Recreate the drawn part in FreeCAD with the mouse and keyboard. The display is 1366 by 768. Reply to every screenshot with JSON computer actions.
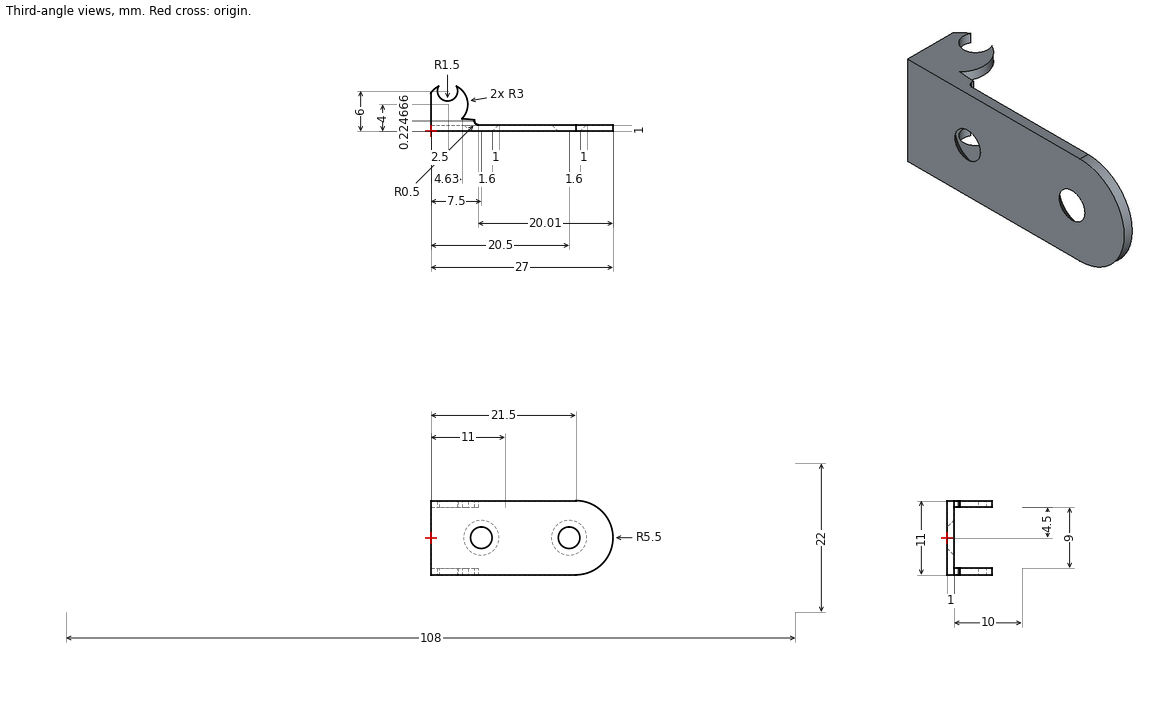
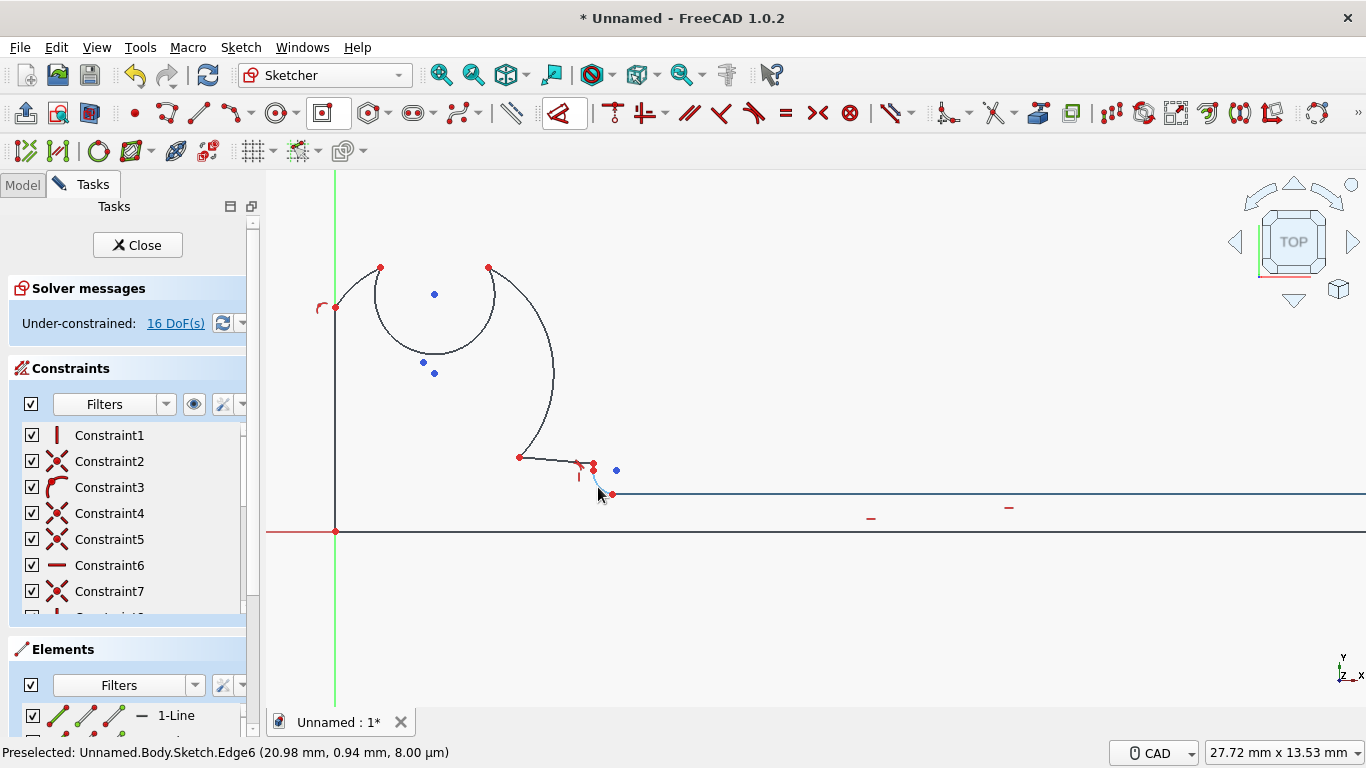
{"action": "left_click", "coordinate": [599, 486]}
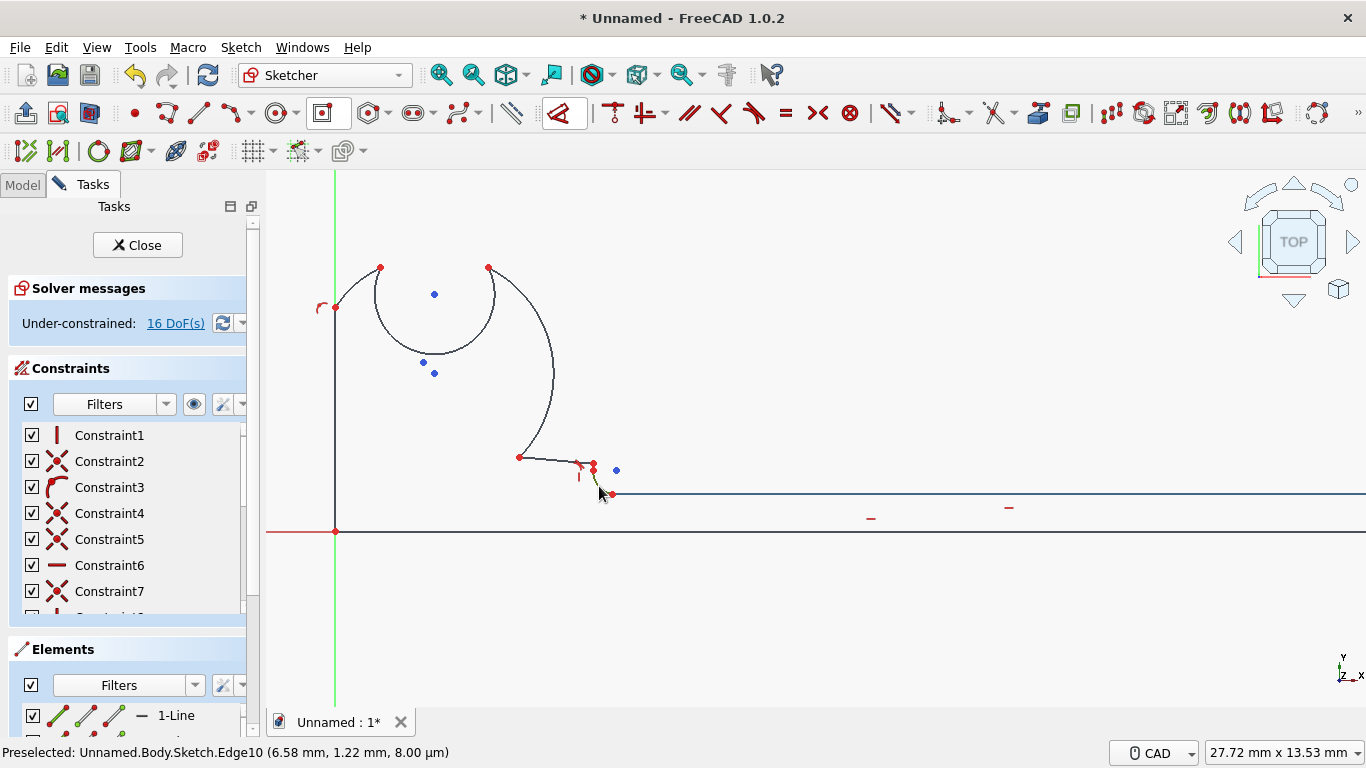
{"action": "key", "text": "t"}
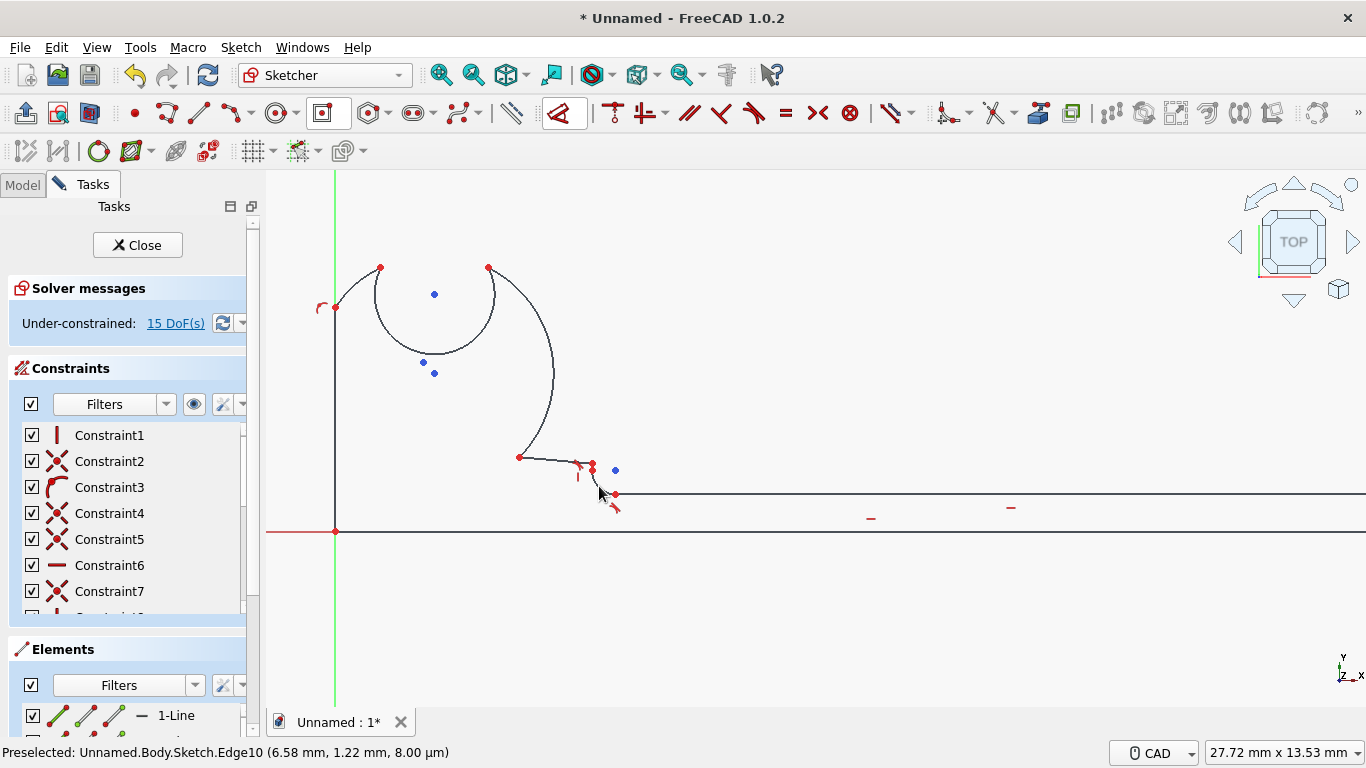
{"action": "left_click", "coordinate": [551, 399]}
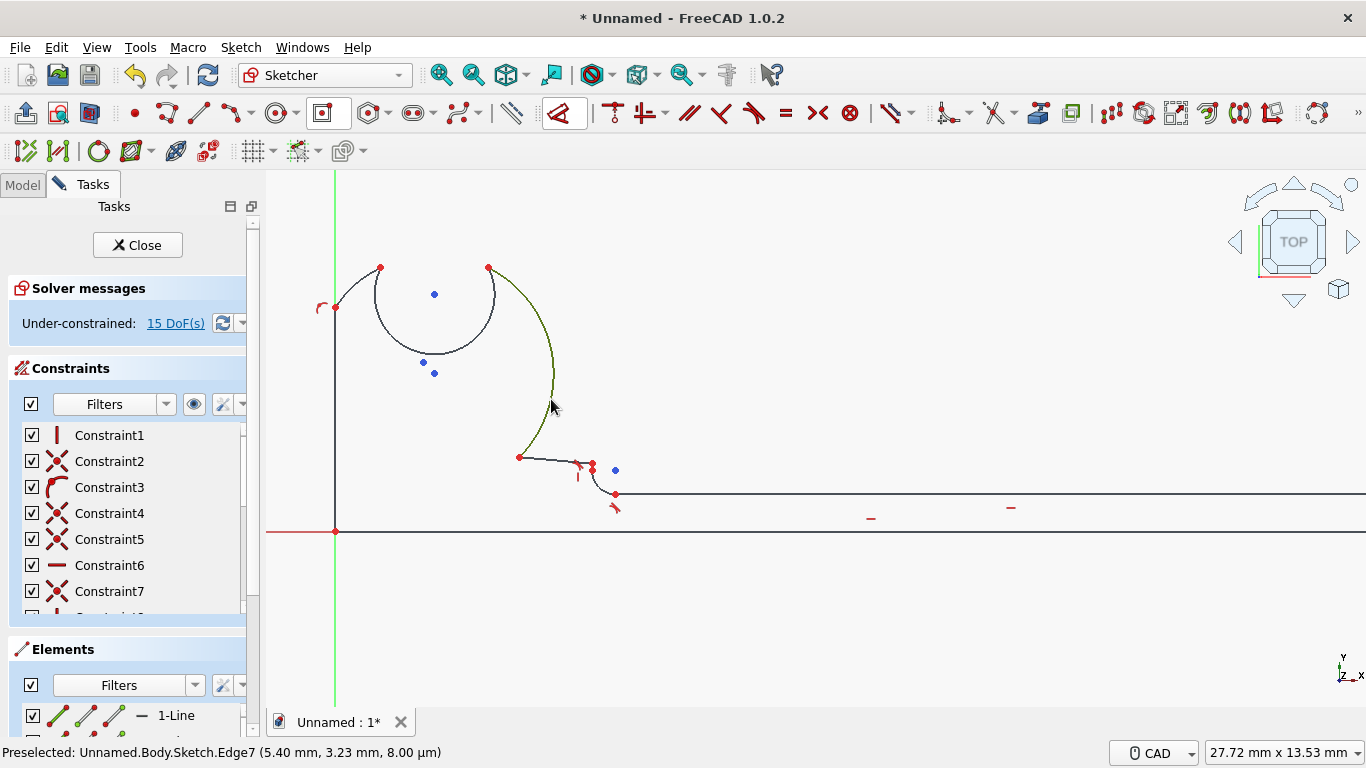
{"action": "left_click", "coordinate": [365, 277]}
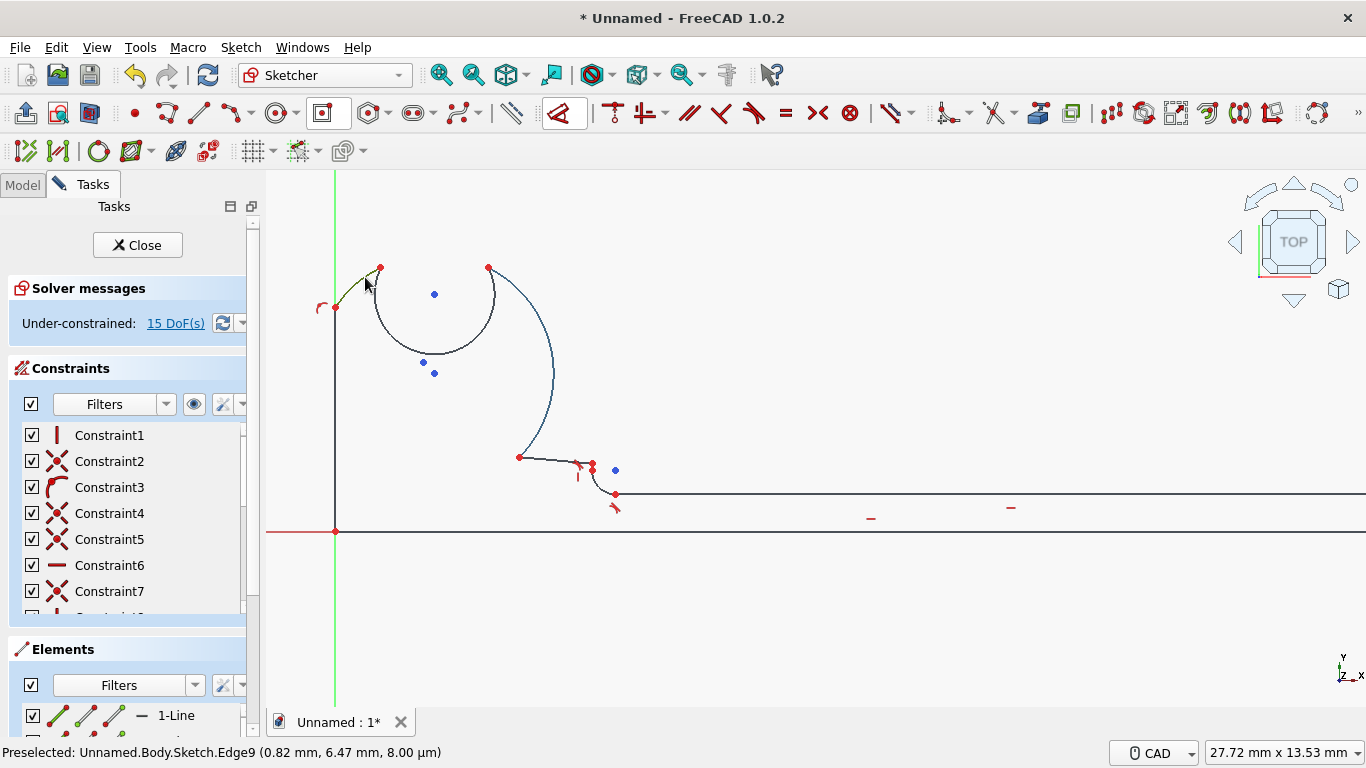
{"action": "key", "text": "c"}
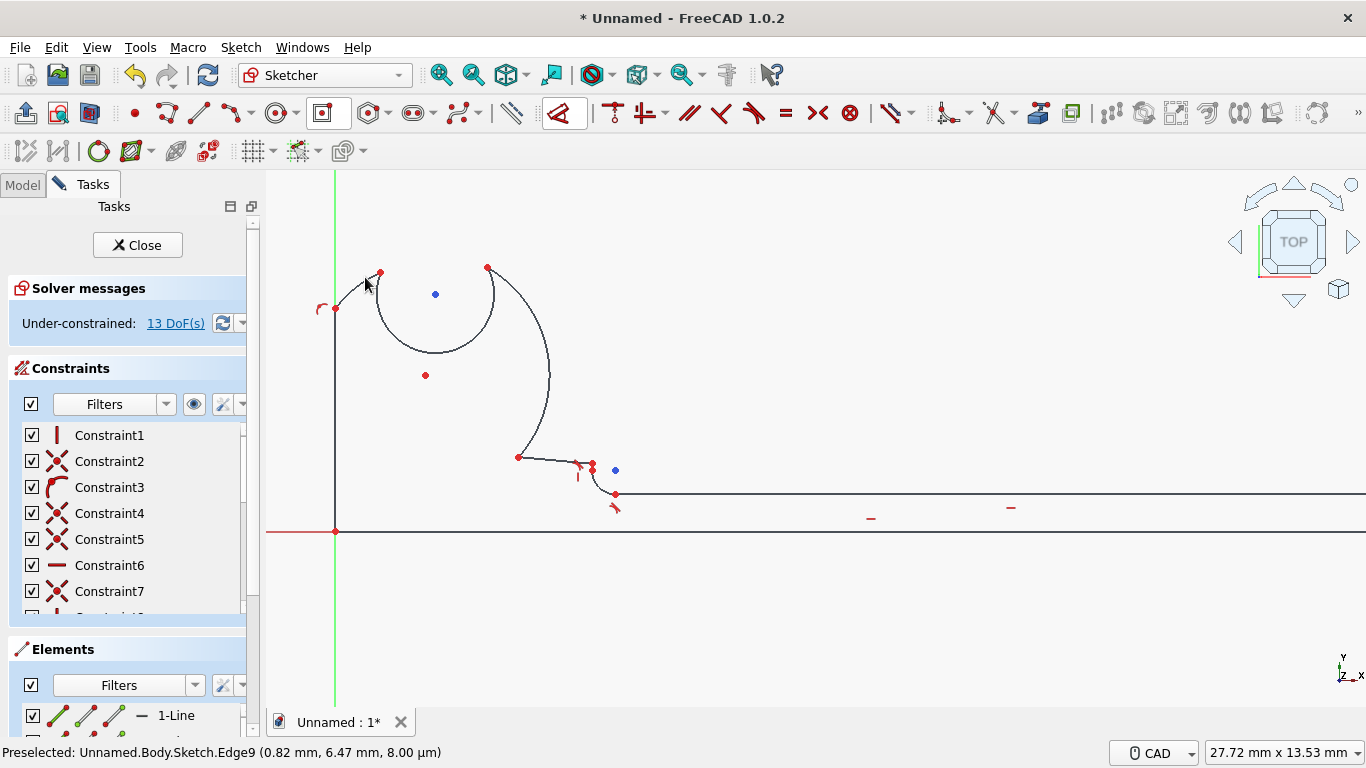
{"action": "left_click", "coordinate": [547, 399]}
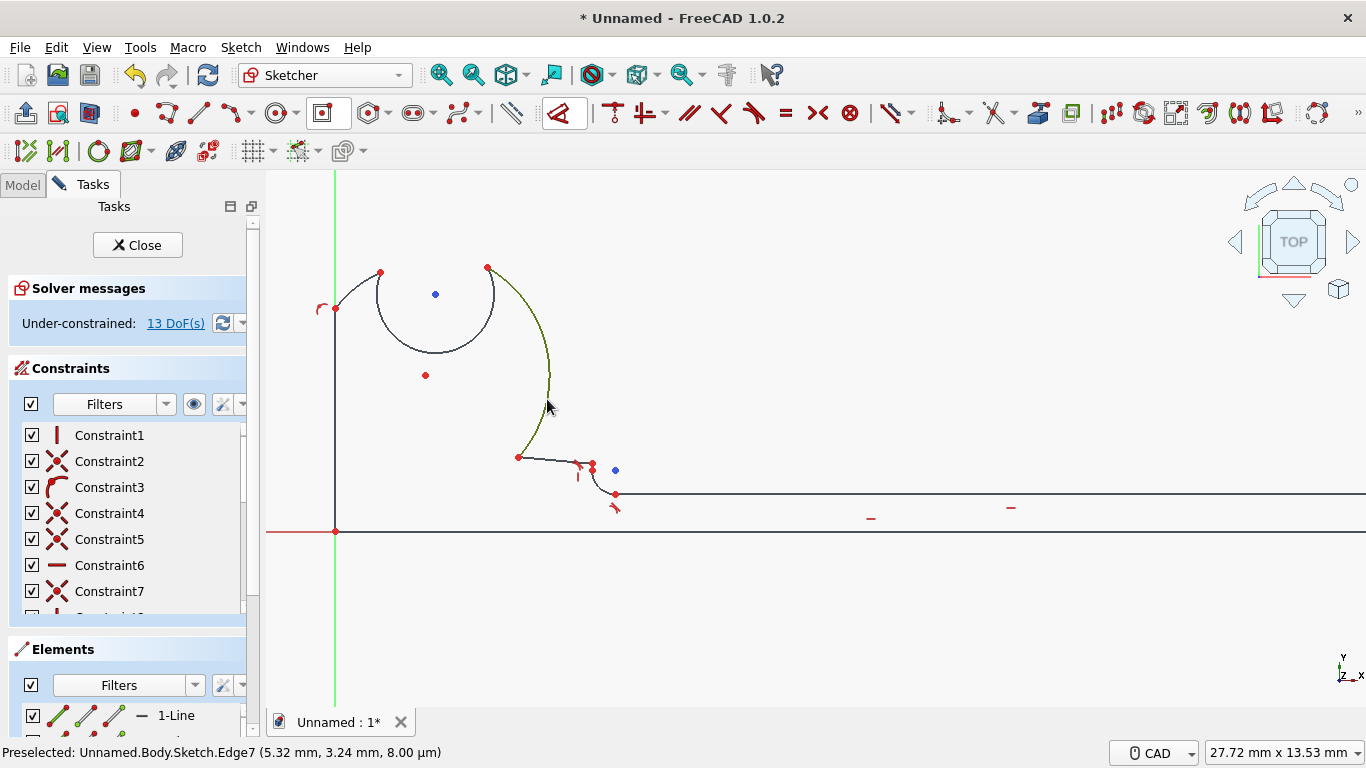
{"action": "left_click", "coordinate": [365, 281]}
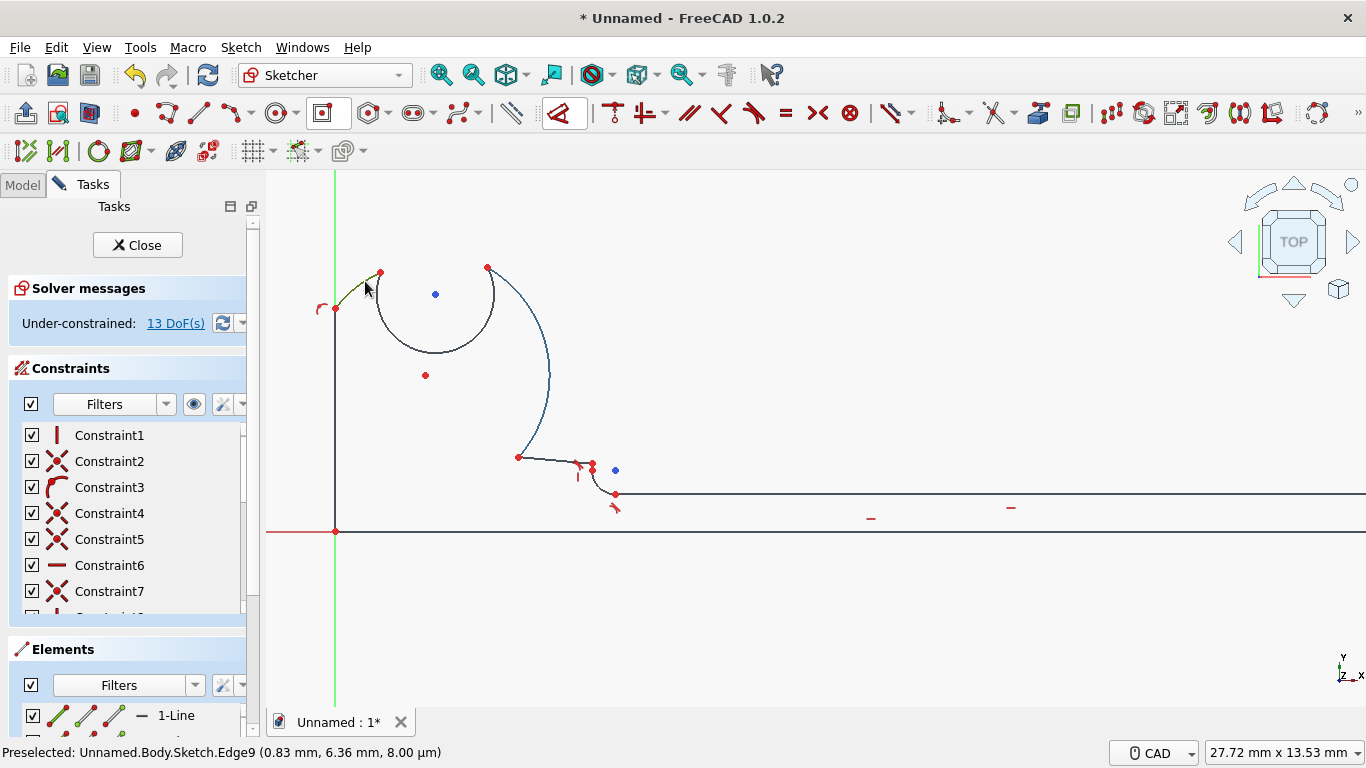
{"action": "key", "text": "e"}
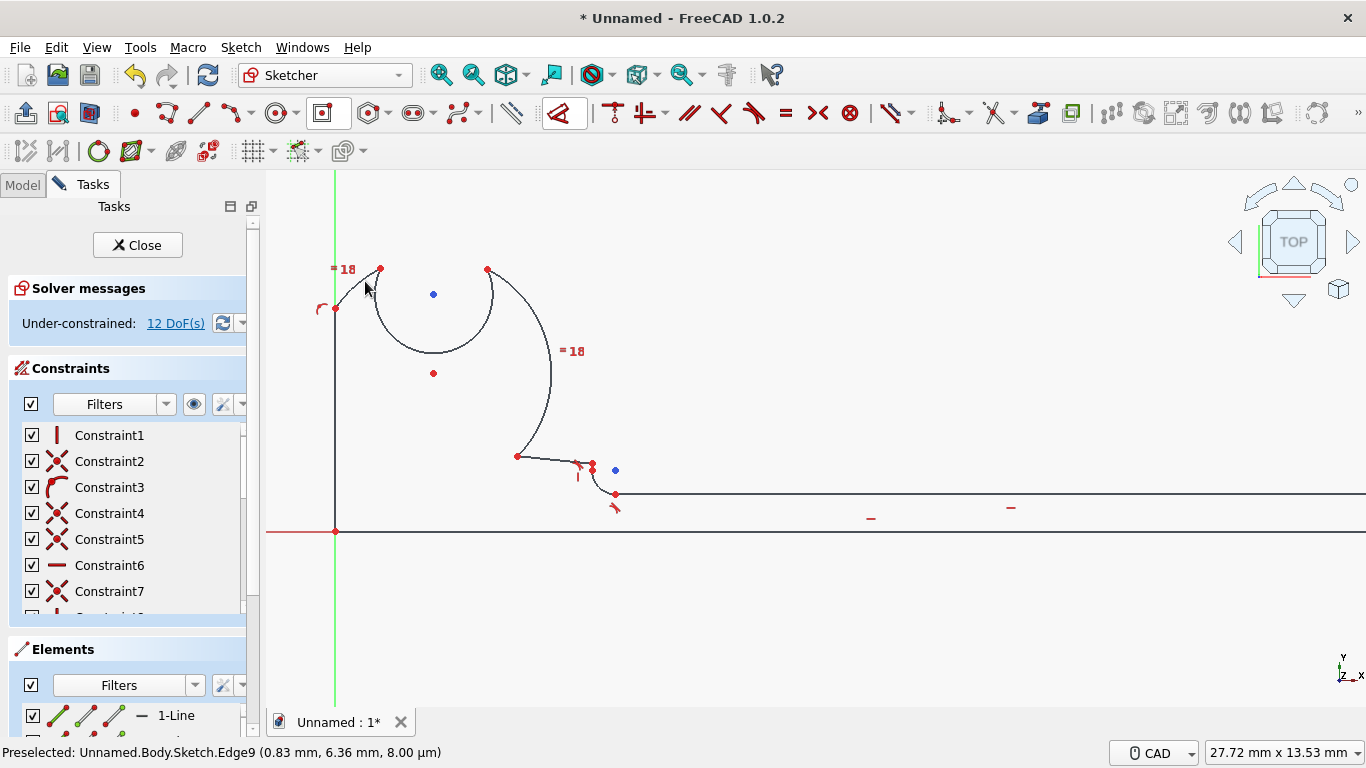
{"action": "key", "text": "d"}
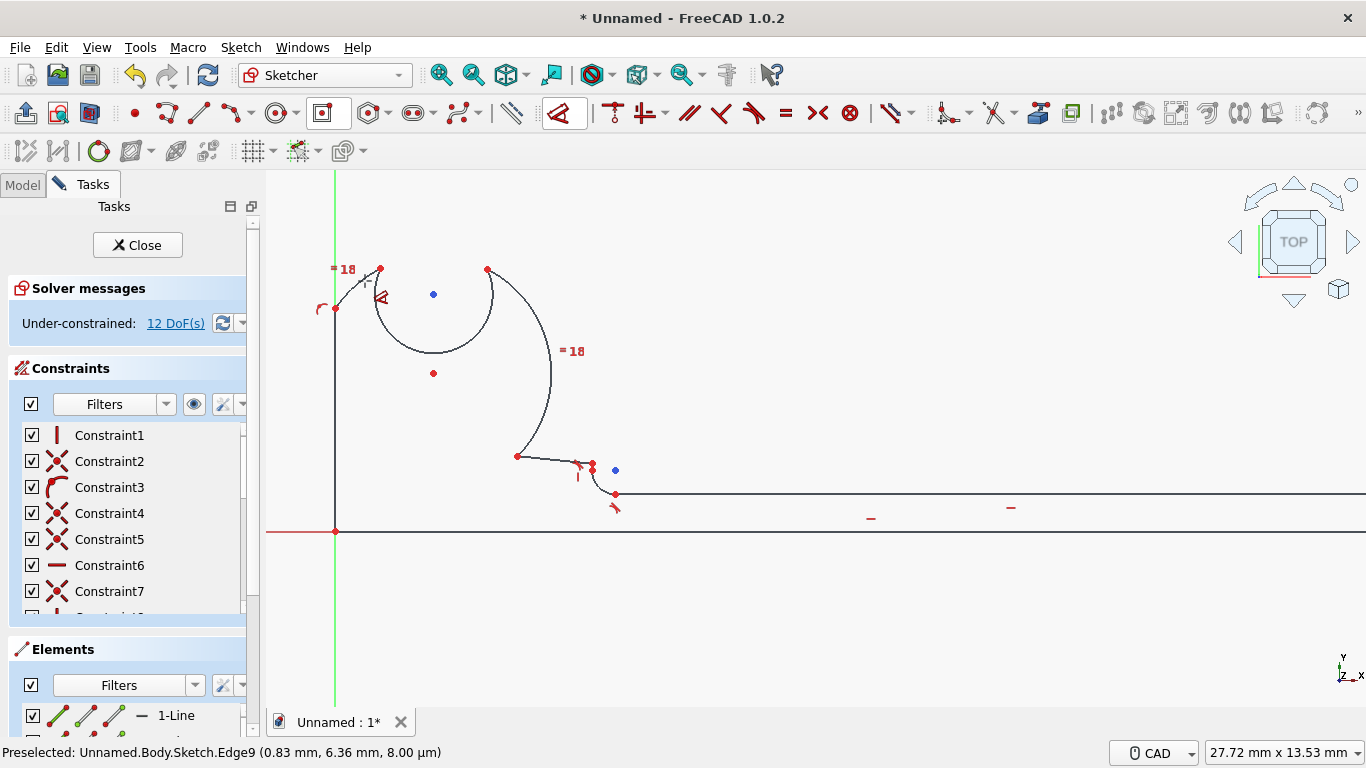
{"action": "left_click", "coordinate": [549, 399]}
{"action": "left_click", "coordinate": [580, 406]}